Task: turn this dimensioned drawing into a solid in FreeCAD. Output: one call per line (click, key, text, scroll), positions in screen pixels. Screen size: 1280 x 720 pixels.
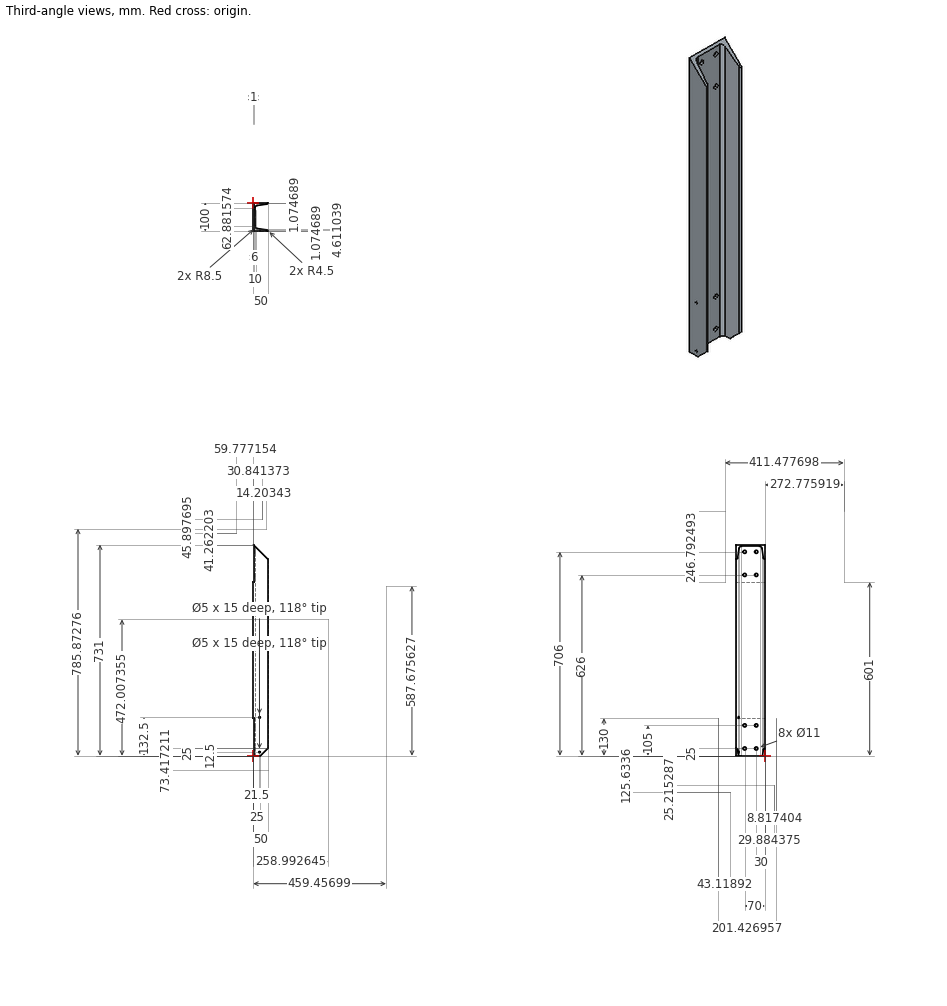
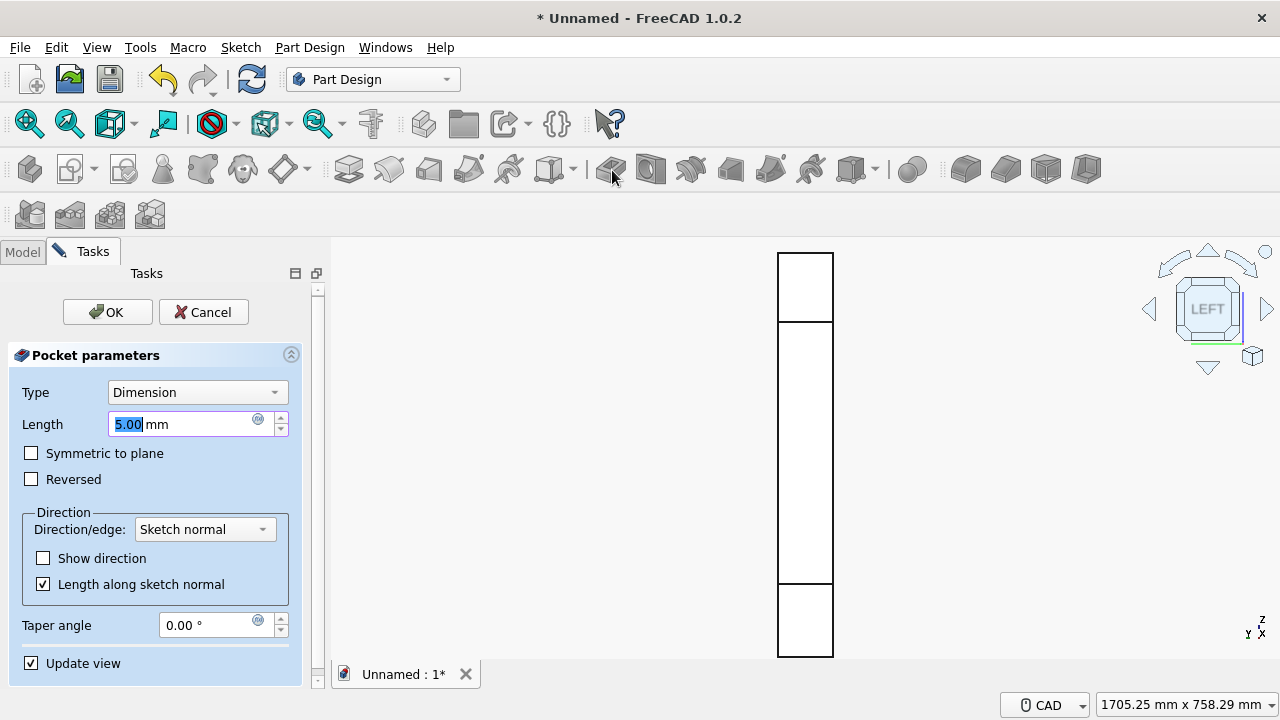
text(1)
key(Tab)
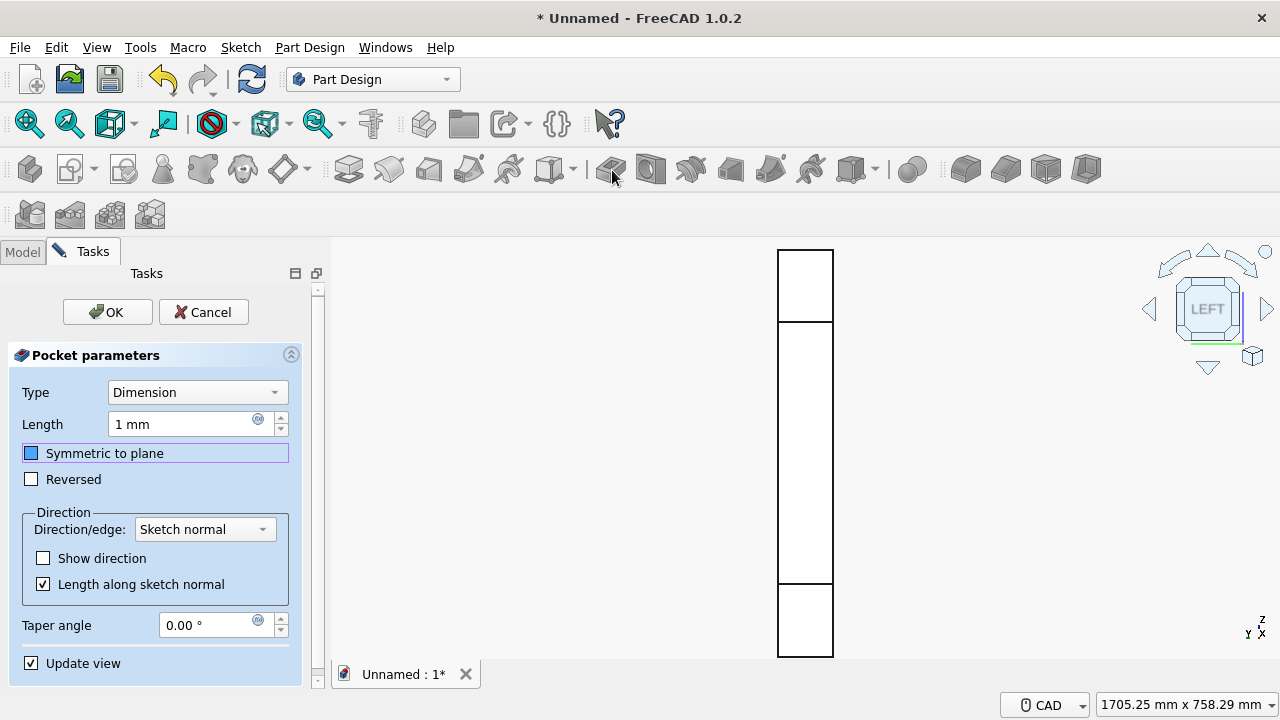
click(108, 312)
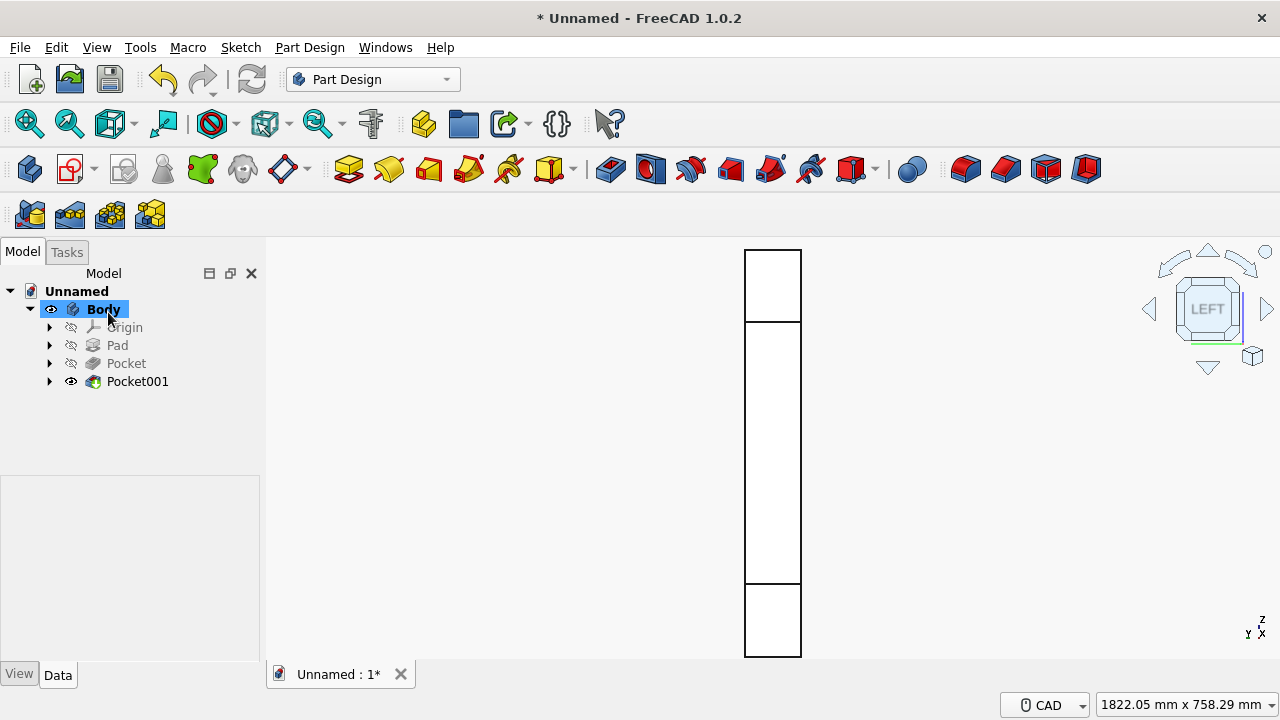
click(773, 620)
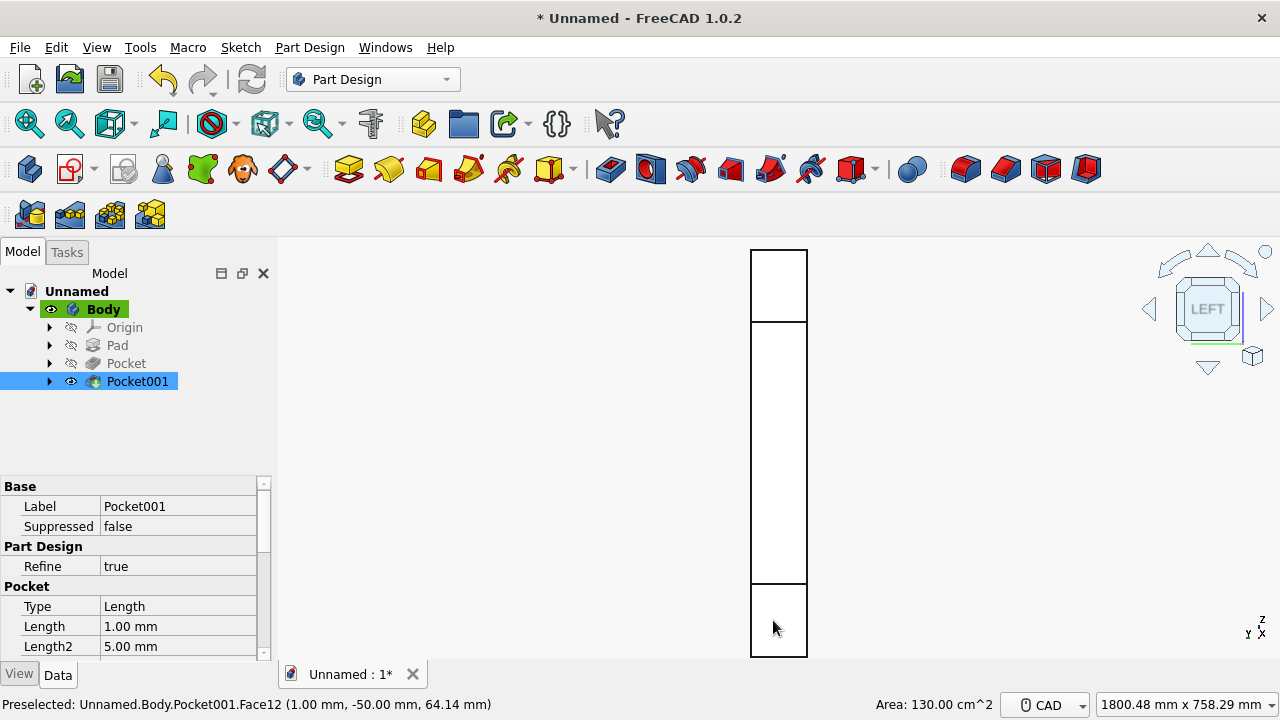
click(70, 170)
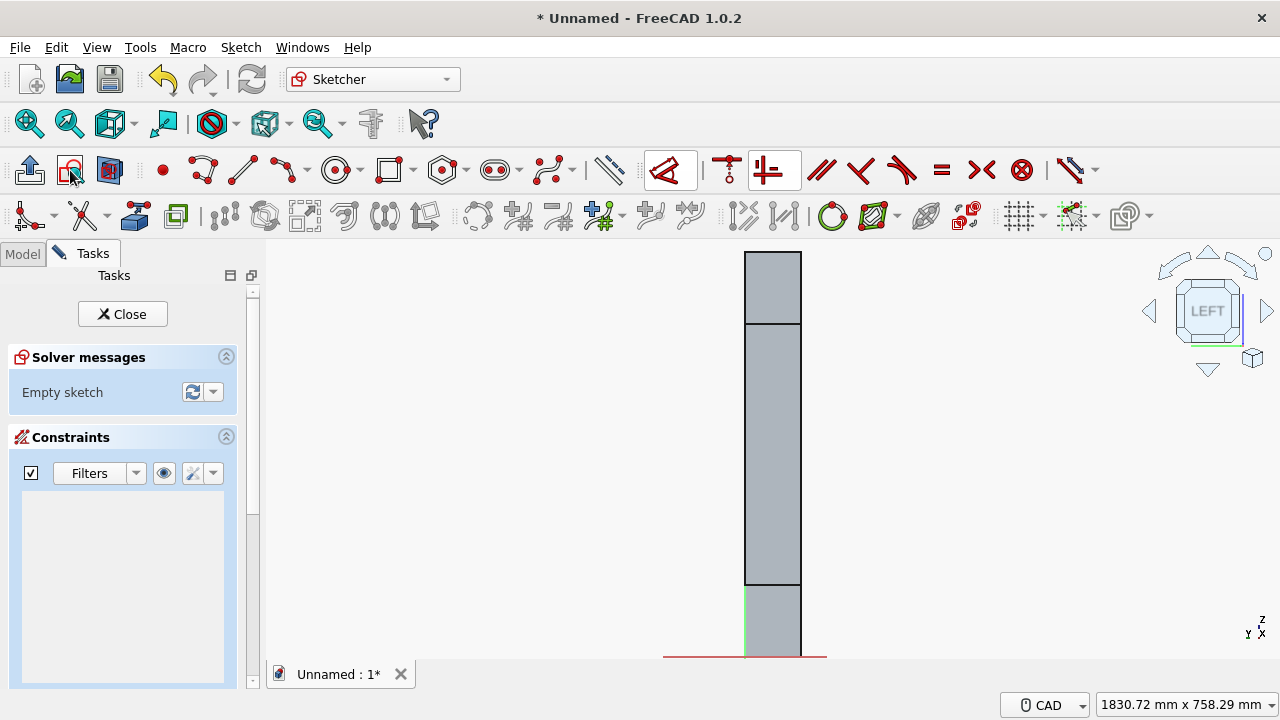
scroll(579, 427, down, 2)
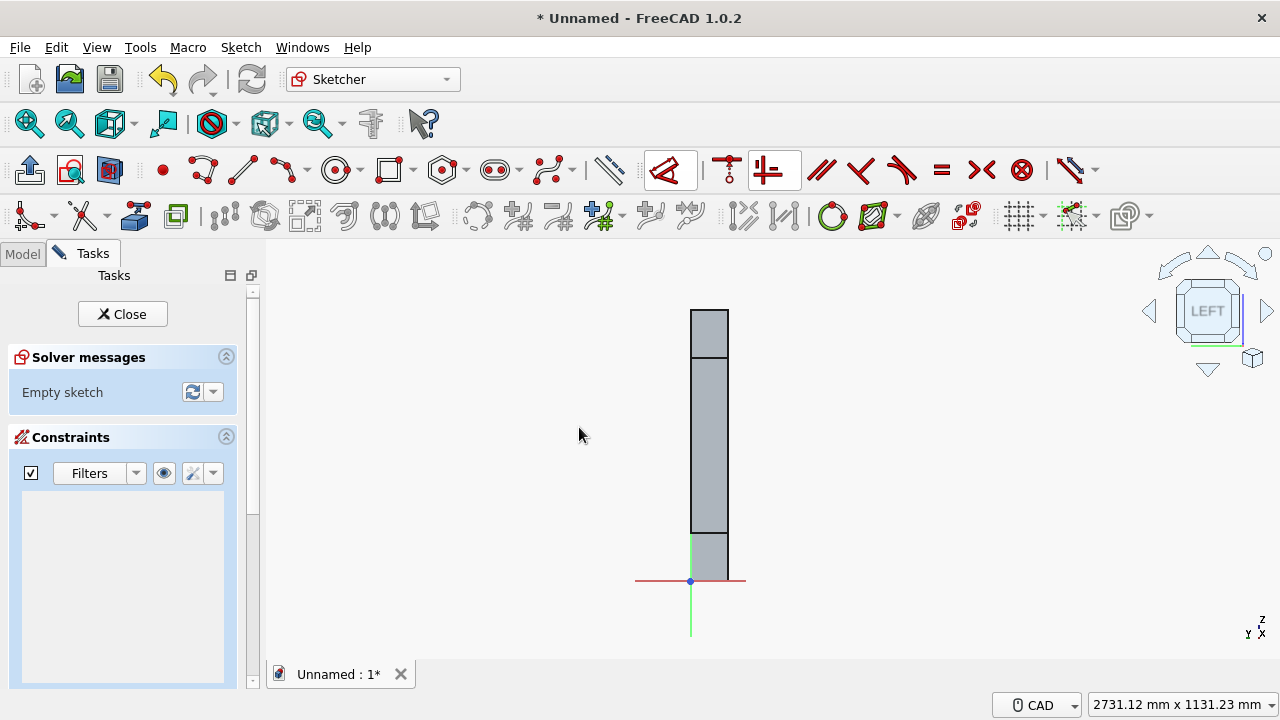
key(g)
key(c)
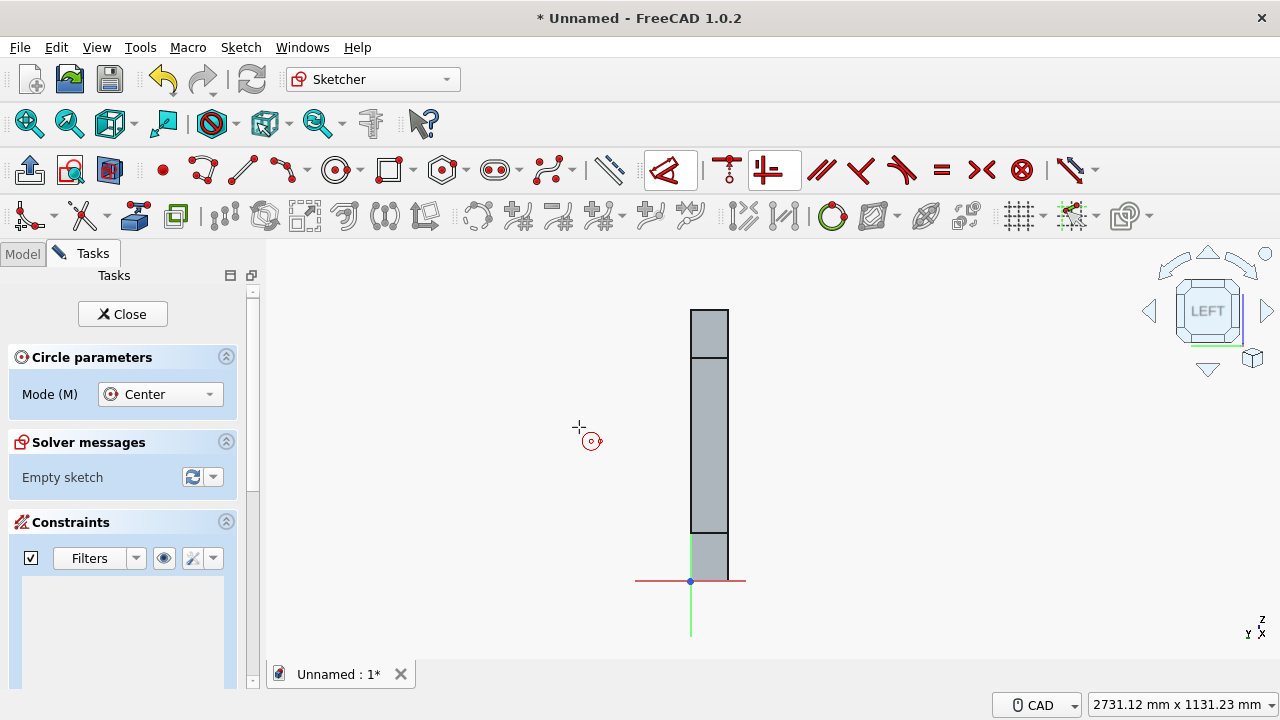
scroll(702, 572, up, 13)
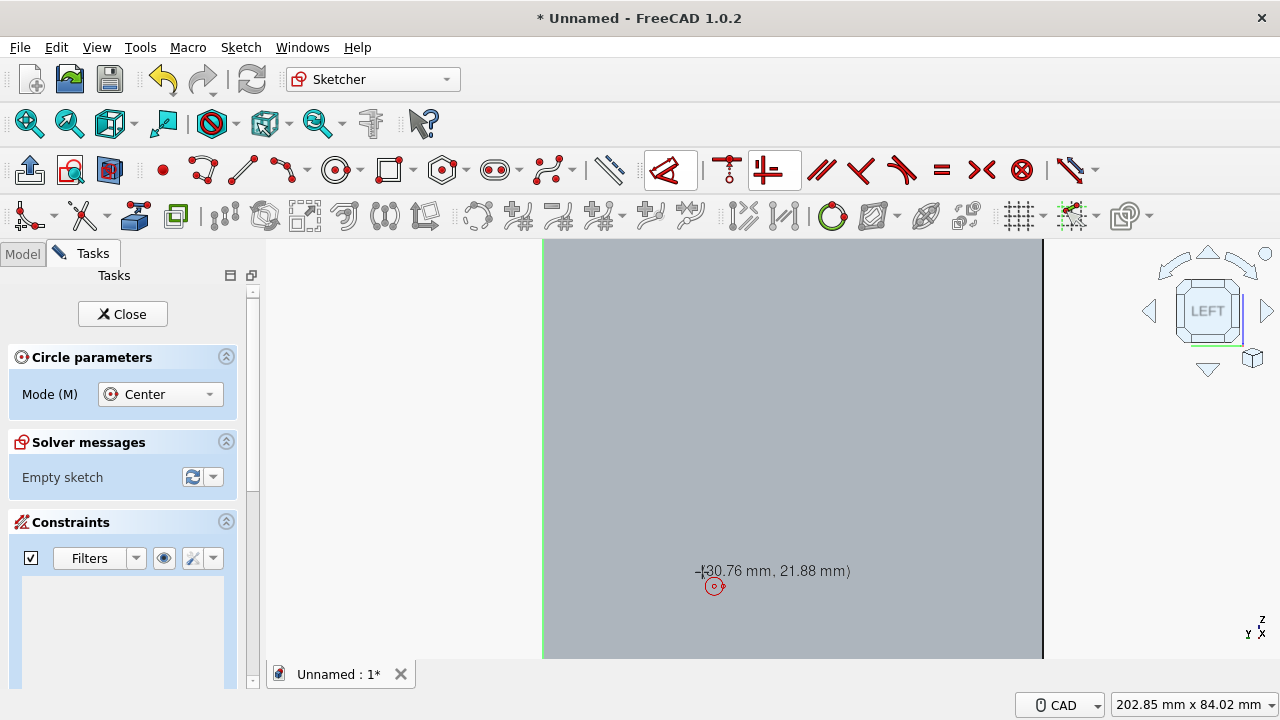
scroll(702, 573, down, 13)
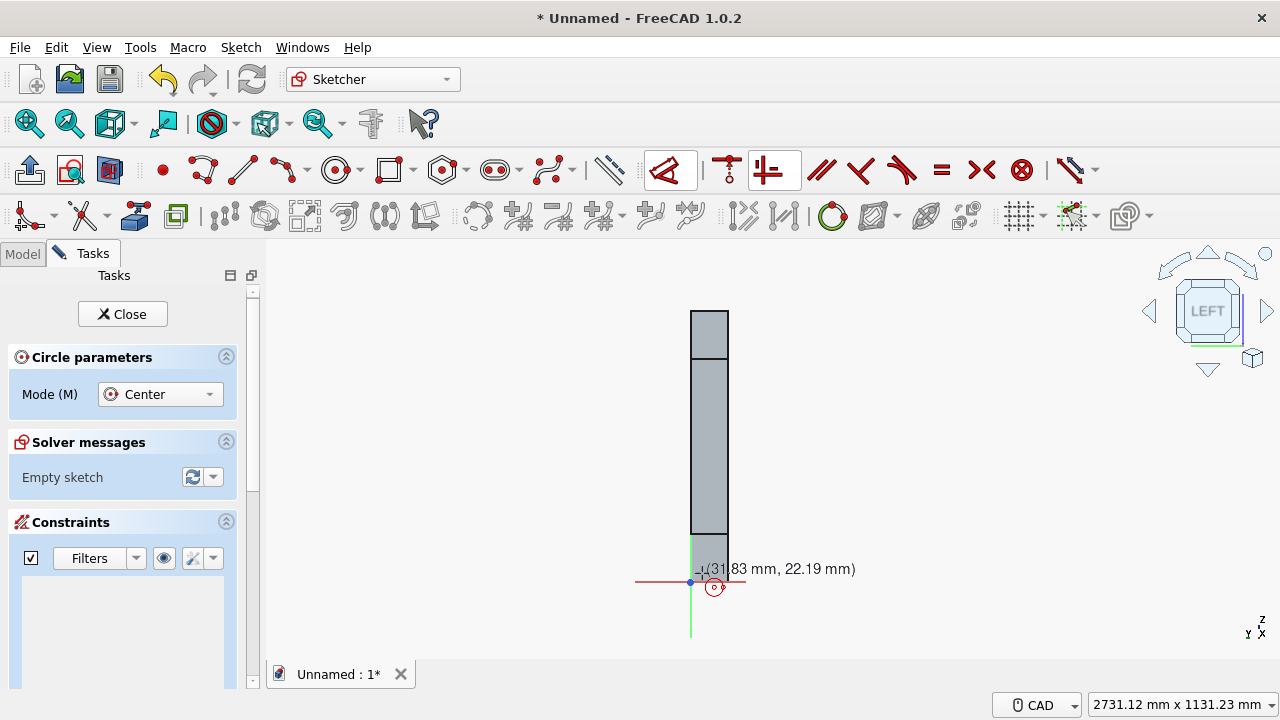
scroll(702, 573, up, 3)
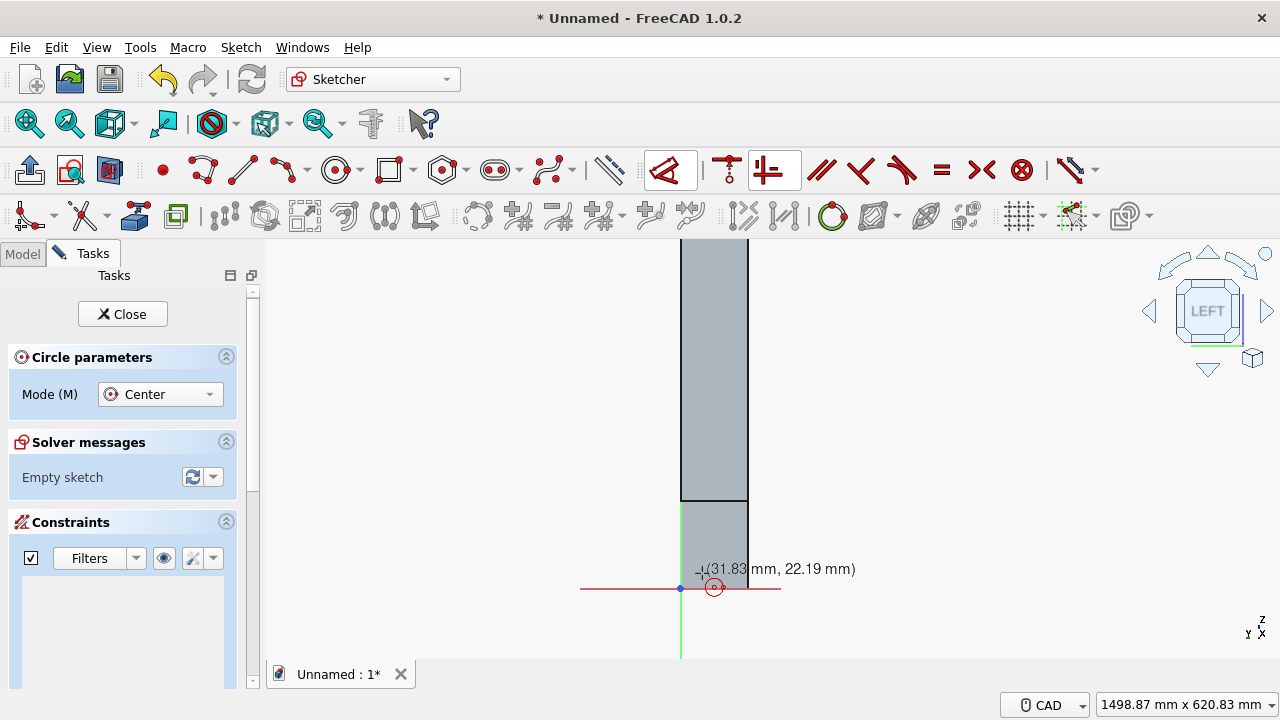
click(701, 572)
move(704, 569)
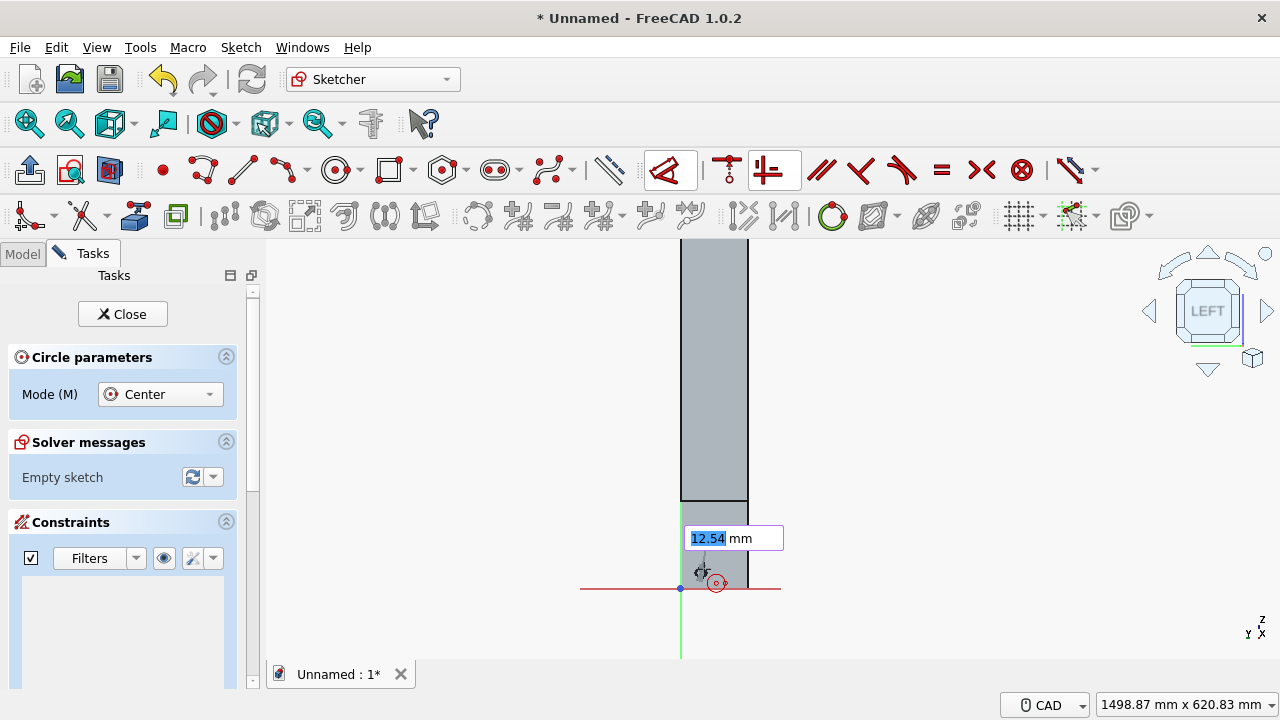
text(11)
key(Return)